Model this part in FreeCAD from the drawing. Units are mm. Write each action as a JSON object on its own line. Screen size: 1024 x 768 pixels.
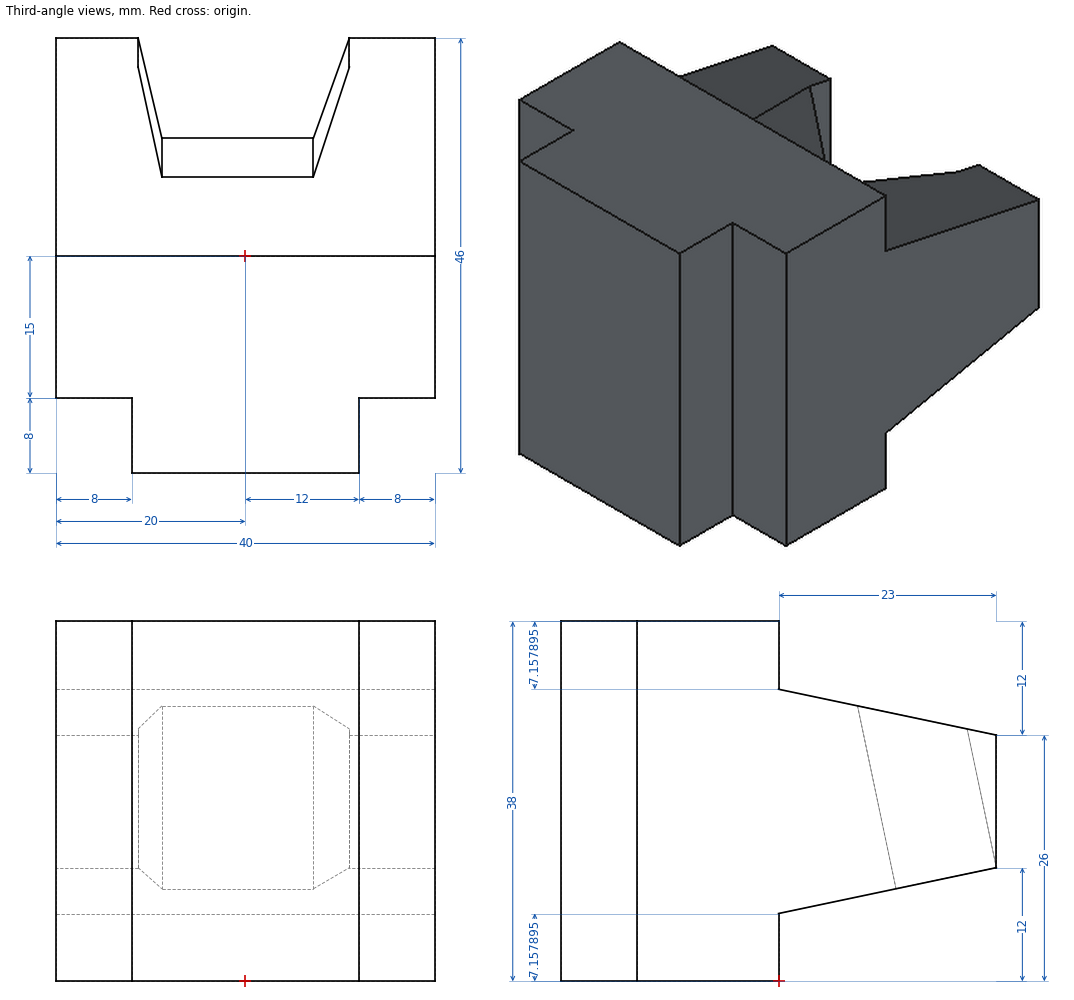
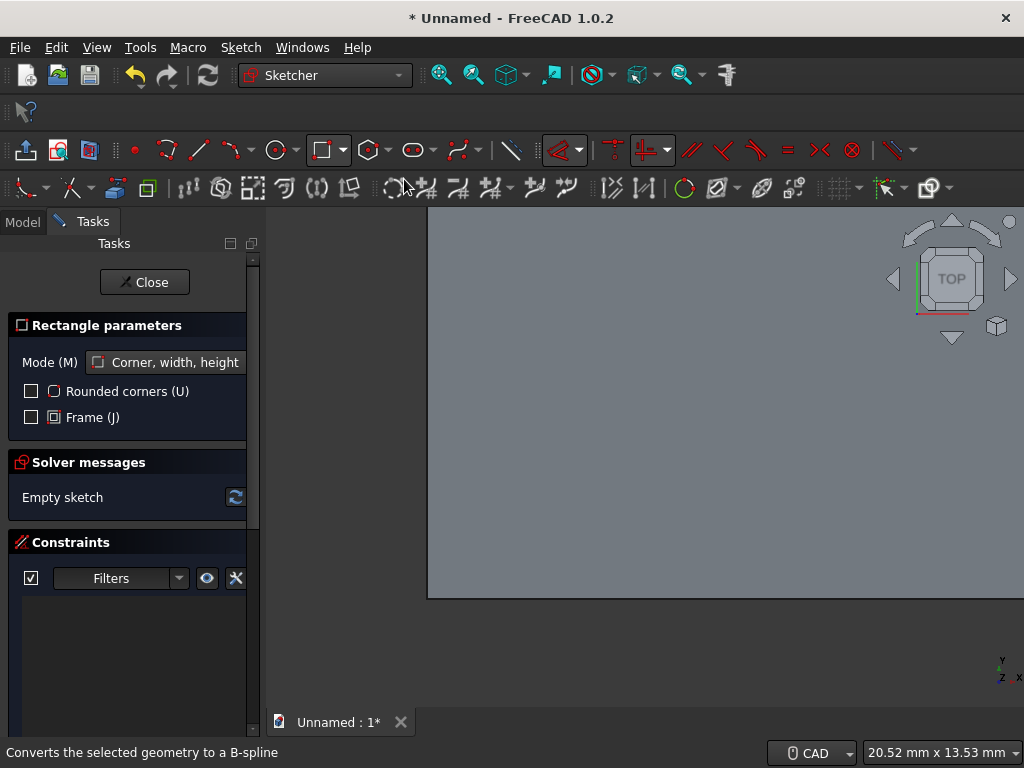
{"action": "left_click", "coordinate": [427, 304]}
{"action": "left_click", "coordinate": [723, 599]}
{"action": "key", "text": "Escape"}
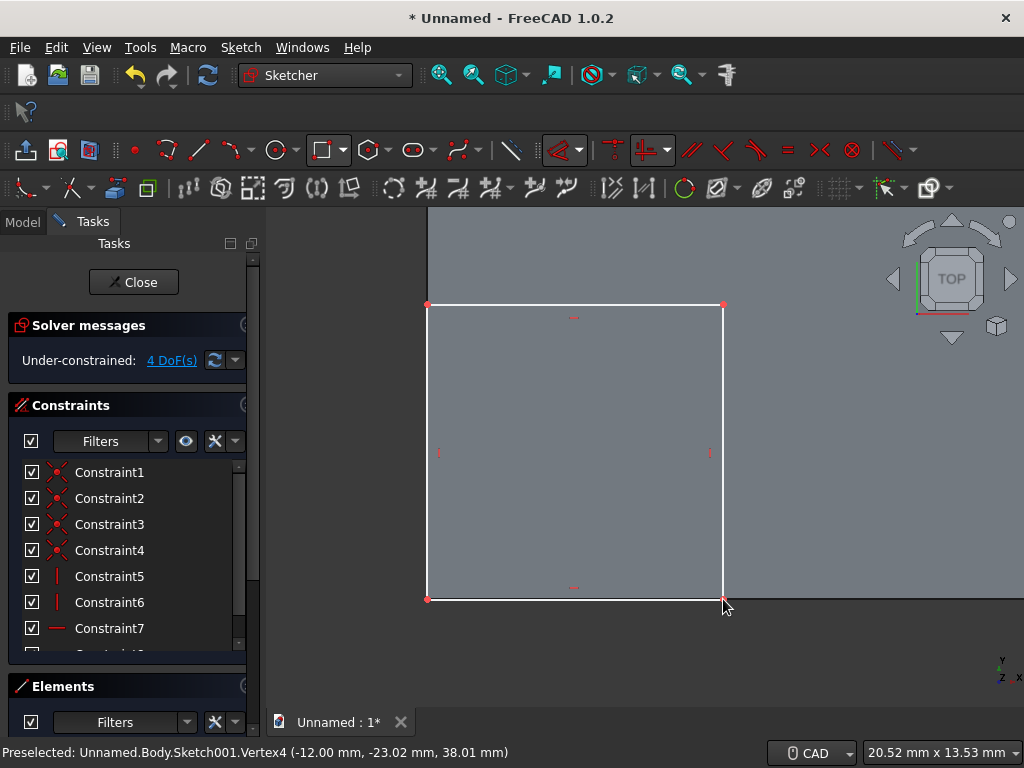
{"action": "left_click", "coordinate": [427, 393]}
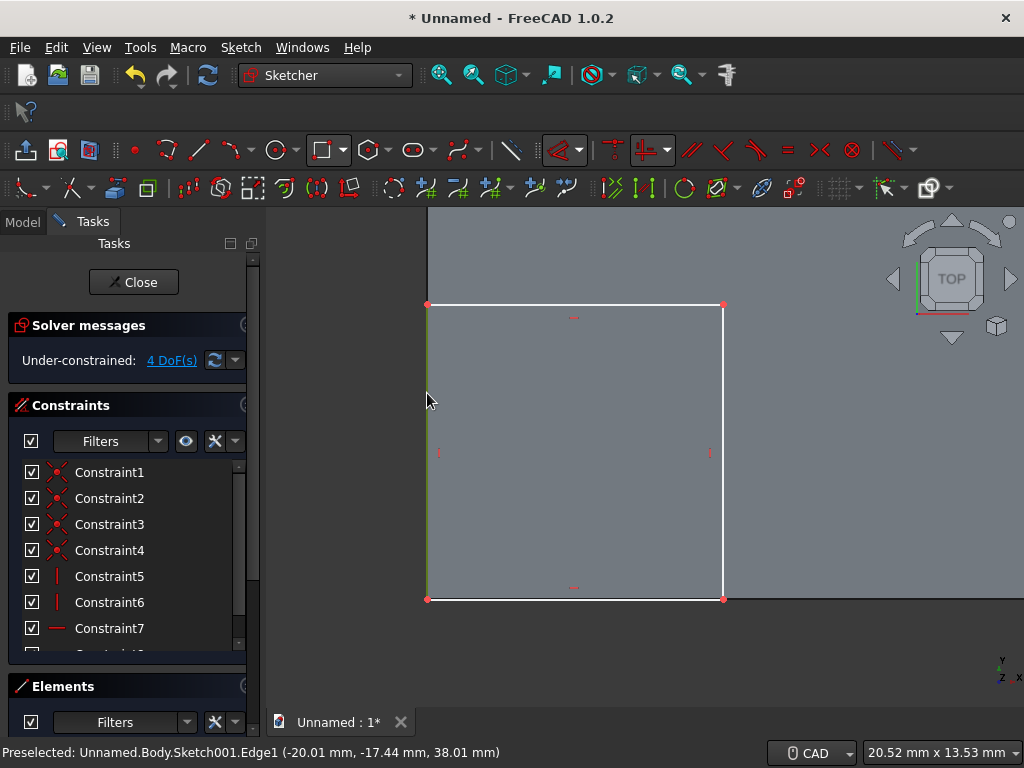
{"action": "left_click", "coordinate": [582, 150]}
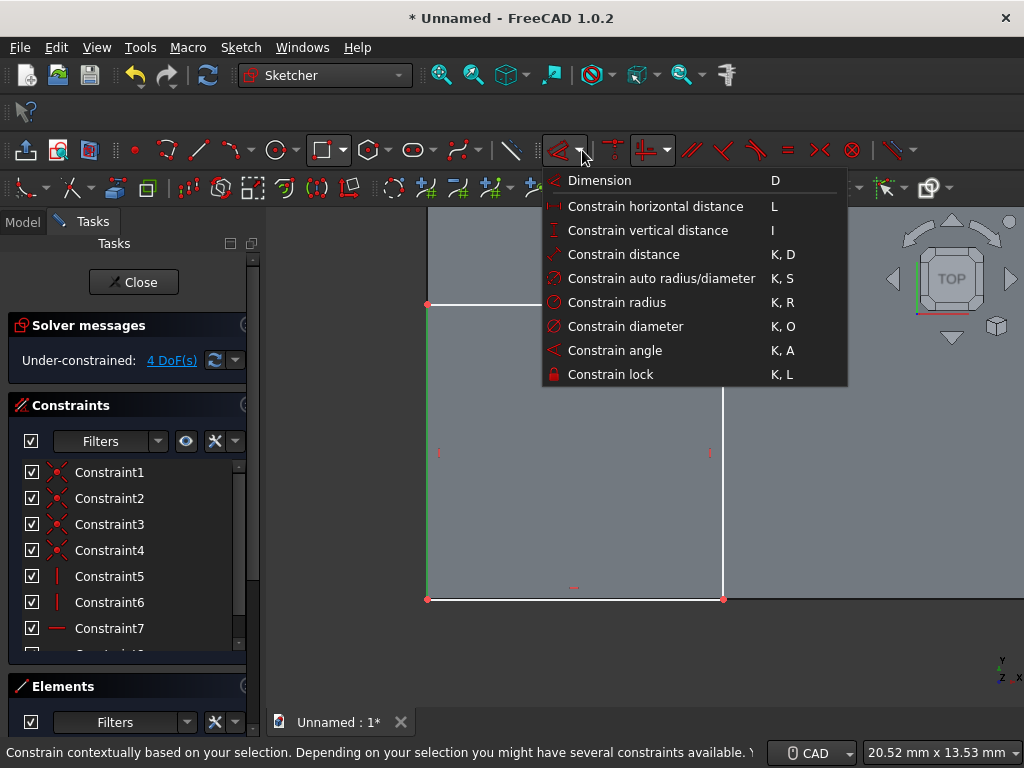
{"action": "left_click", "coordinate": [695, 230]}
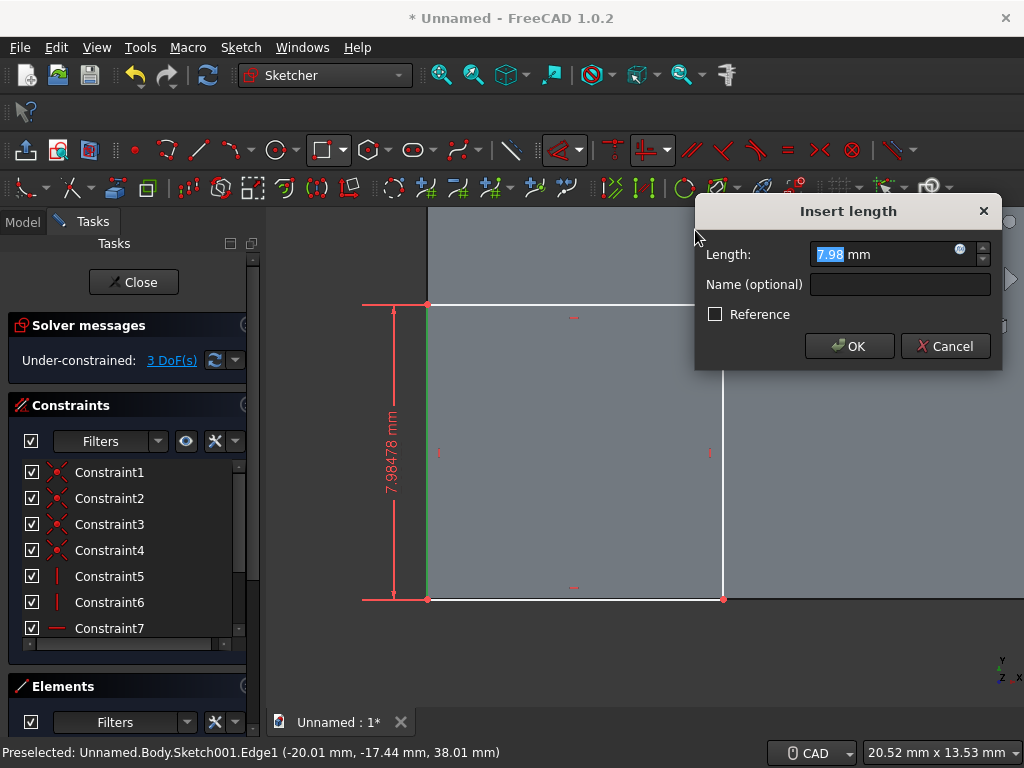
{"action": "type", "text": "8"}
{"action": "key", "text": "Return"}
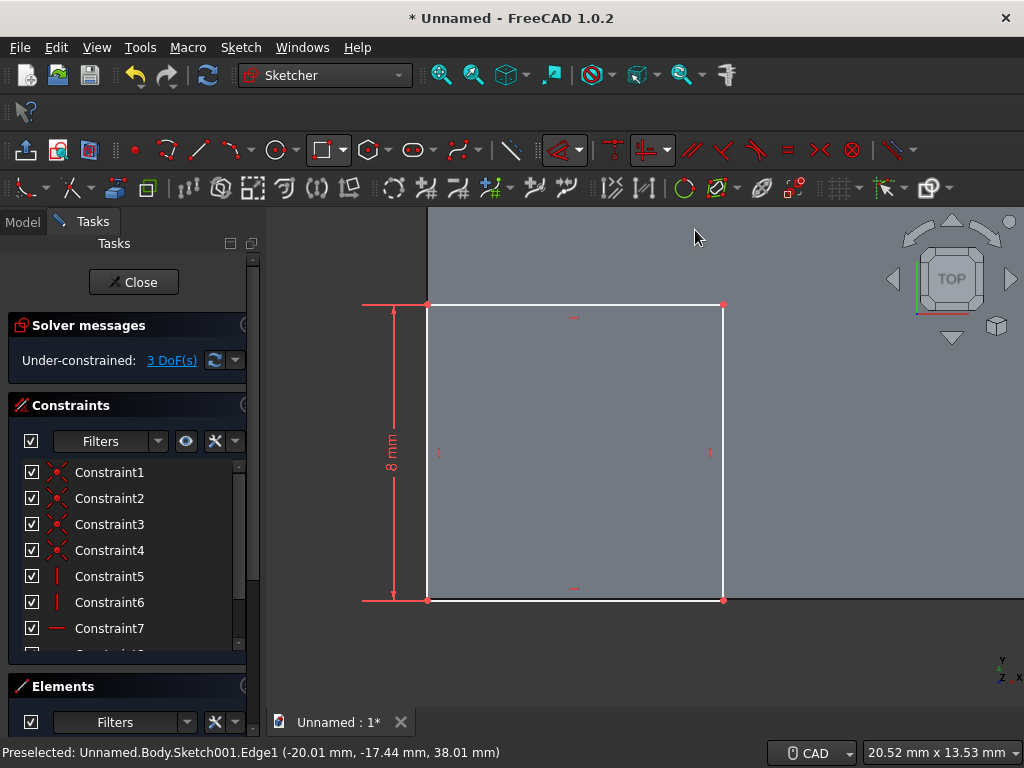
{"action": "left_click", "coordinate": [516, 601]}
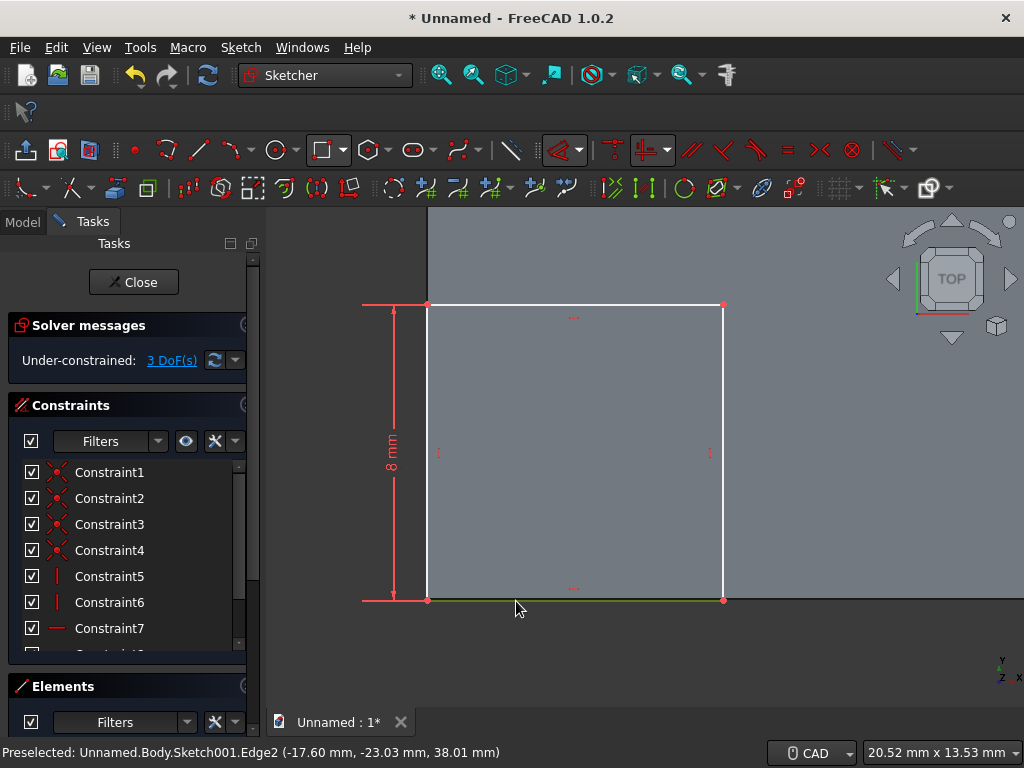
{"action": "key", "text": "l"}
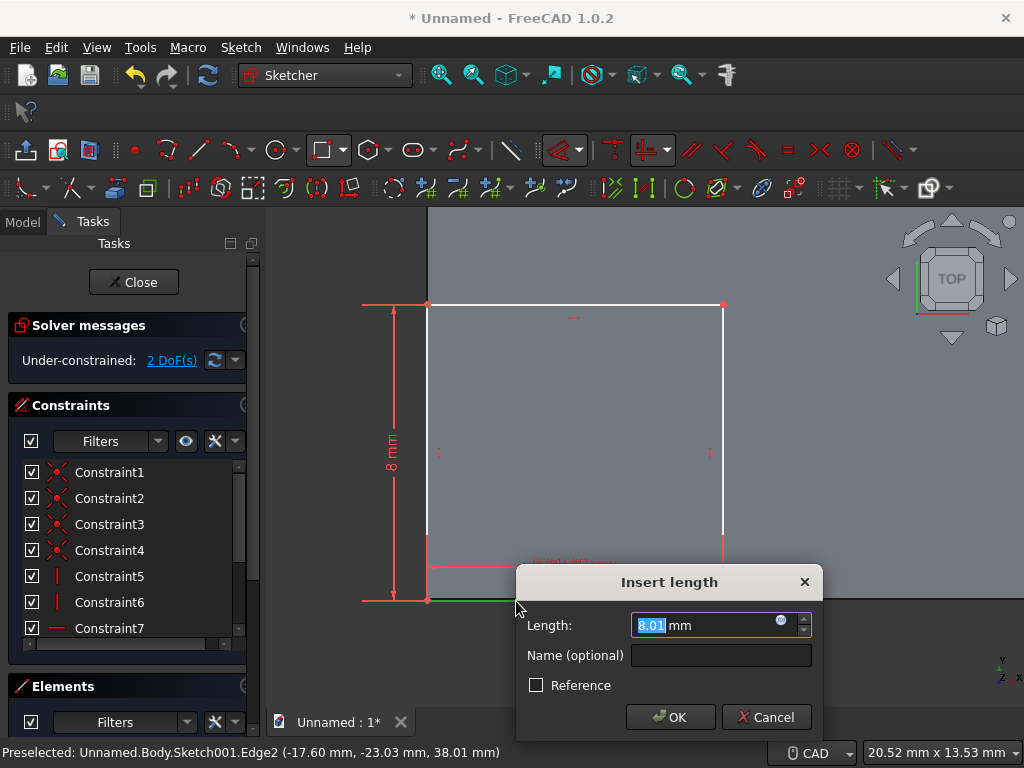
{"action": "type", "text": "8"}
{"action": "key", "text": "Return"}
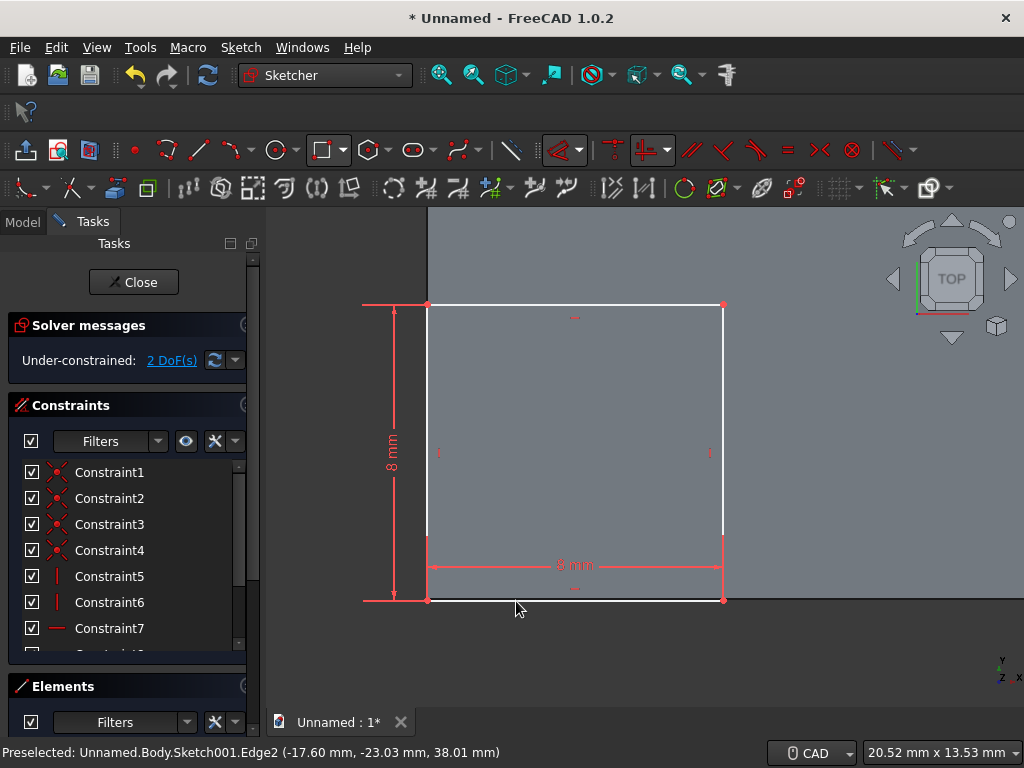
{"action": "left_click", "coordinate": [427, 305]}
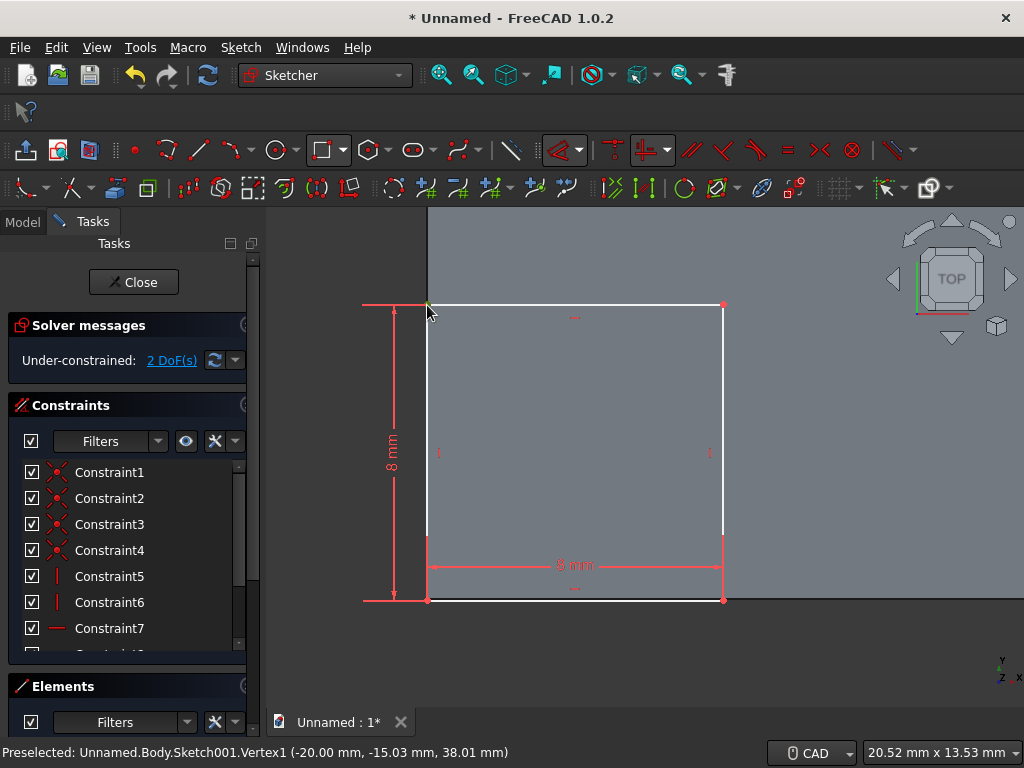
{"action": "left_click", "coordinate": [582, 150]}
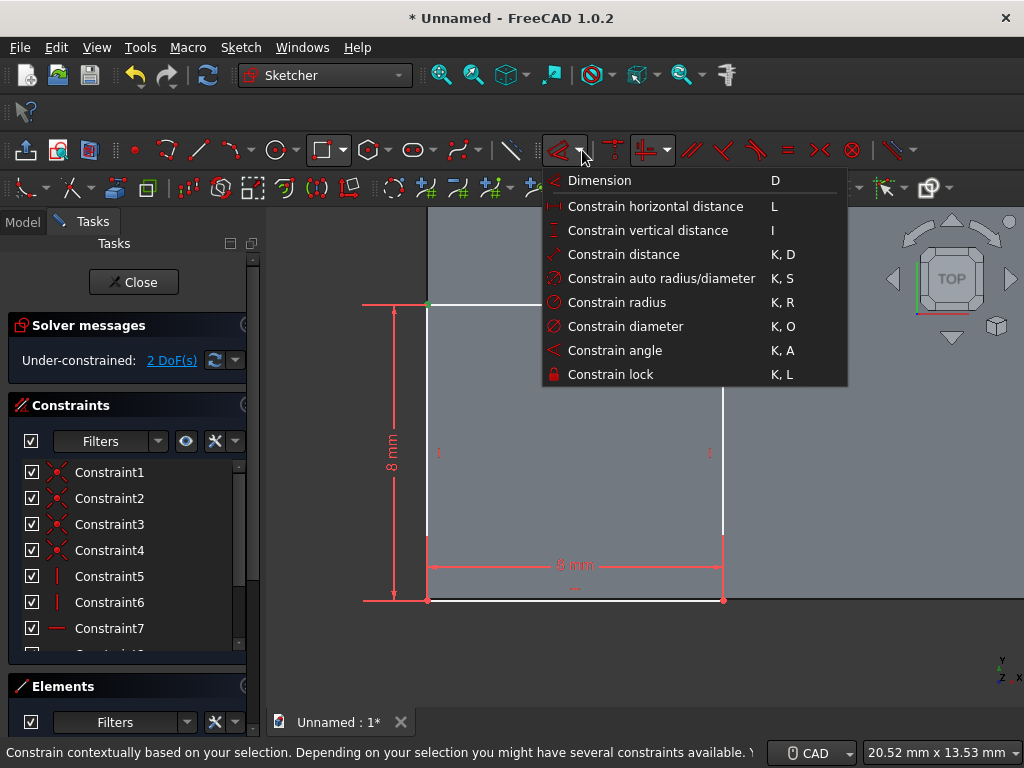
{"action": "left_click", "coordinate": [695, 206]}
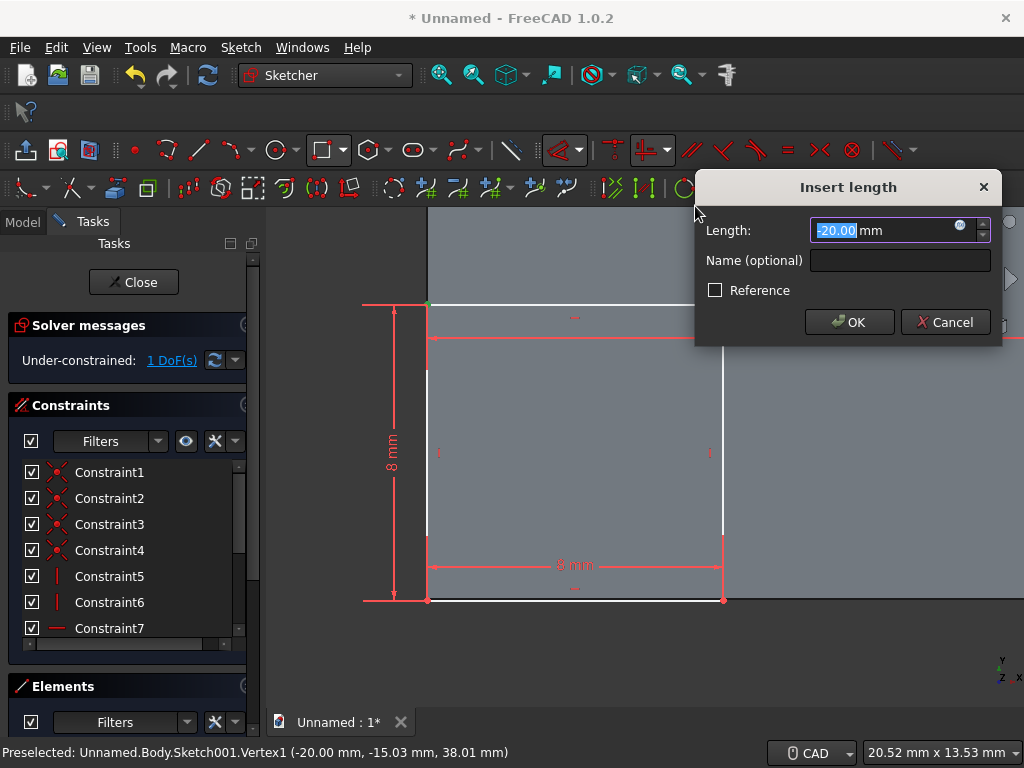
{"action": "type", "text": "-20"}
{"action": "key", "text": "Return"}